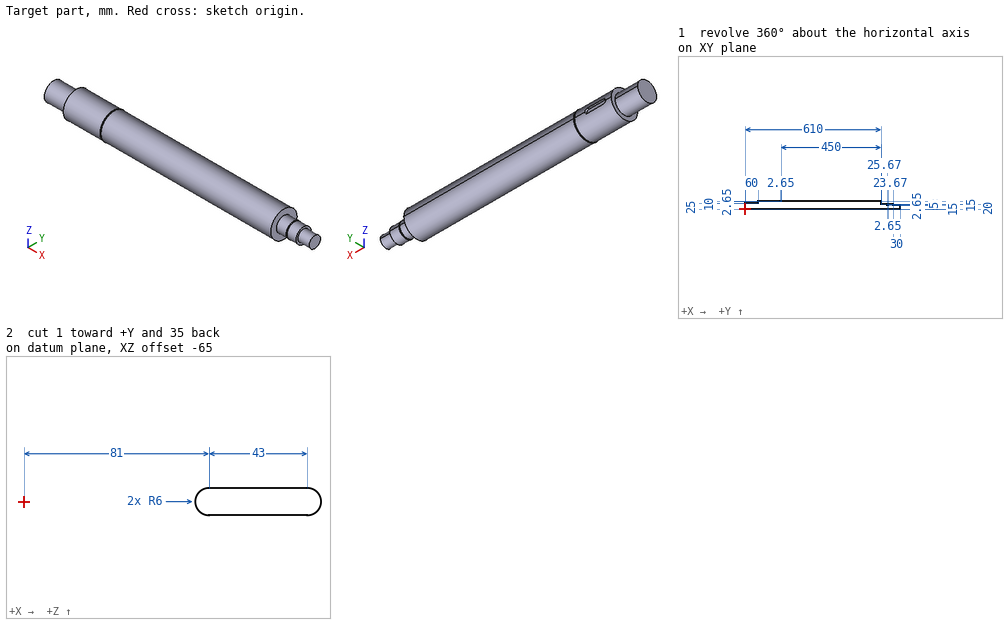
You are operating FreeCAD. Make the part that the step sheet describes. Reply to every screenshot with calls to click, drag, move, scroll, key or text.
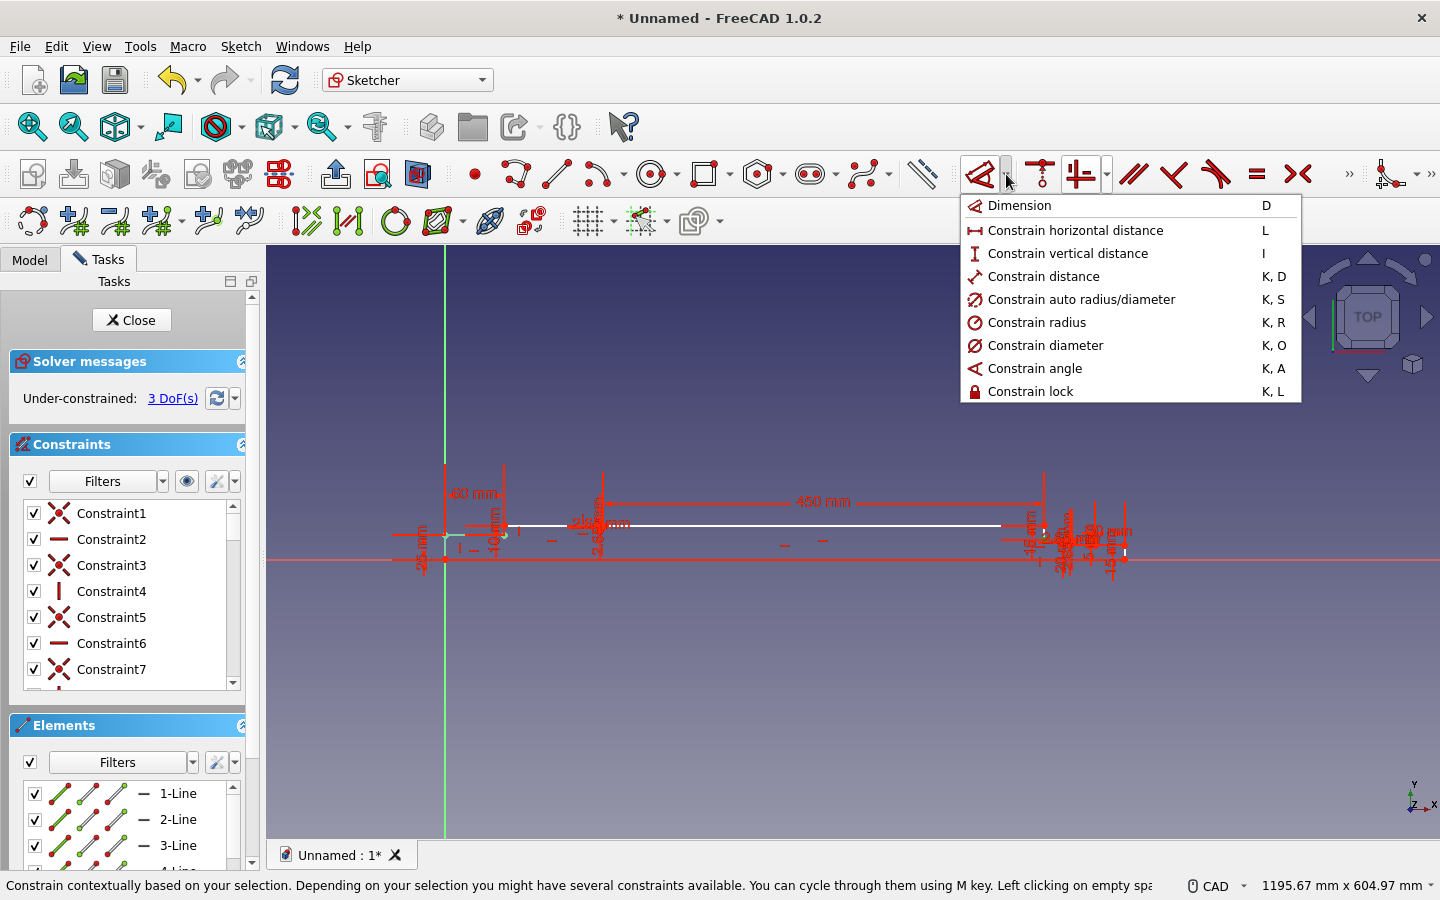
click(1131, 230)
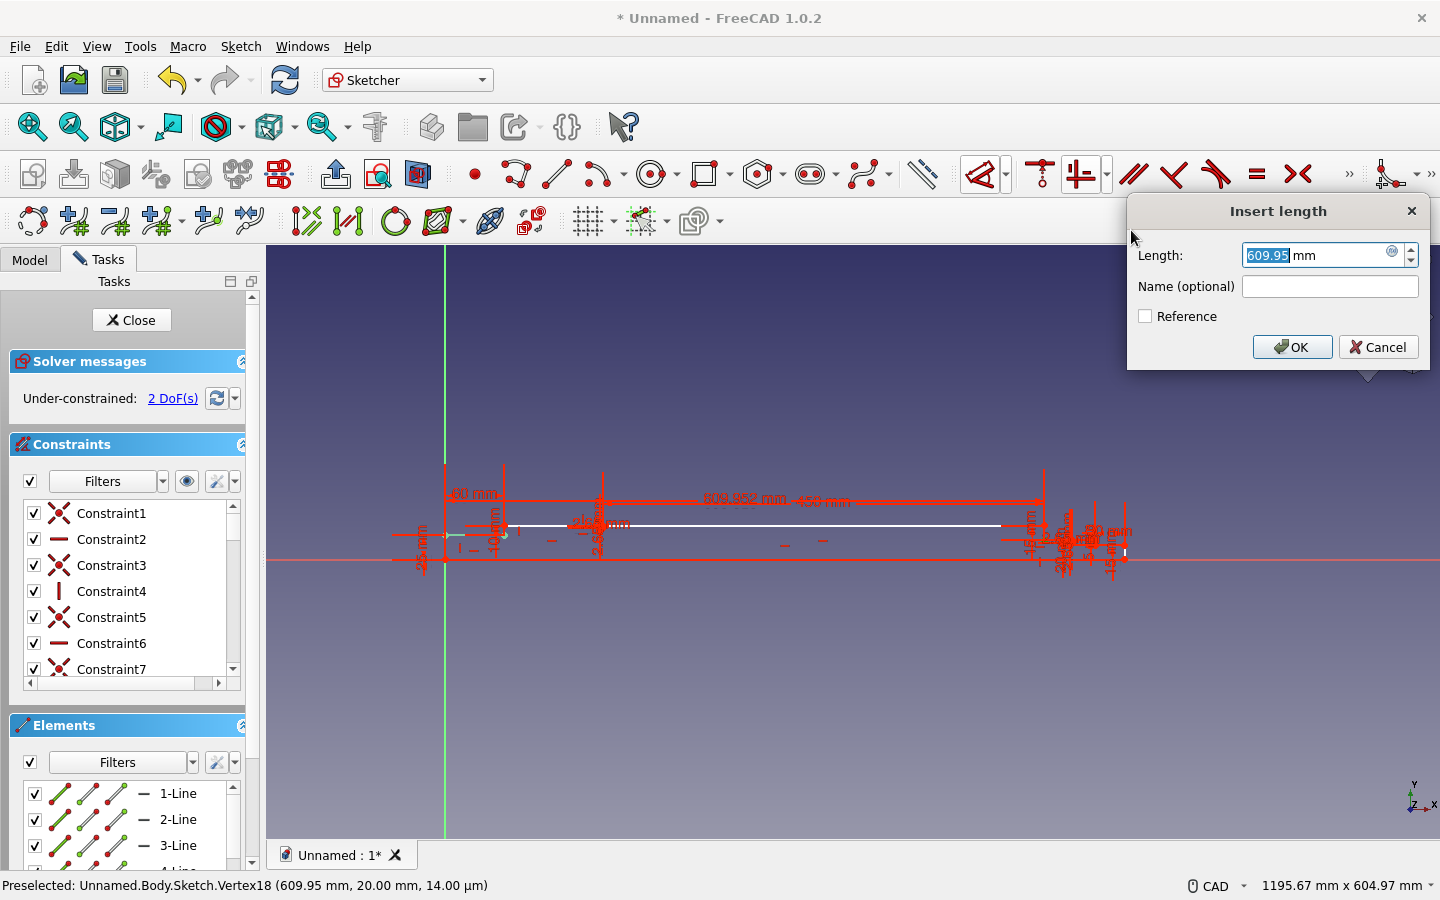
text(610)
key(Return)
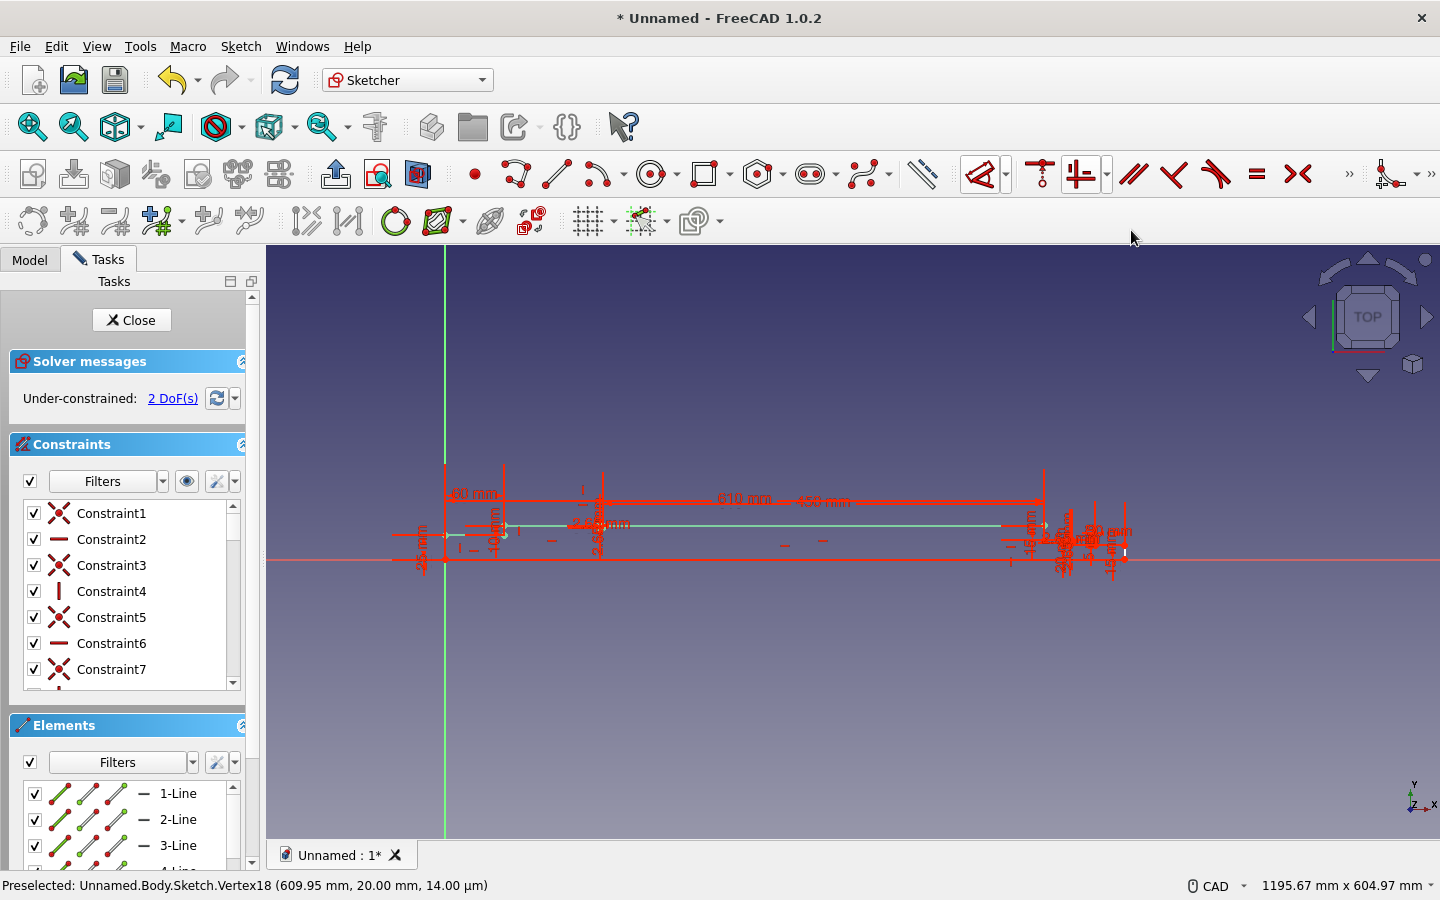
scroll(1086, 540, up, 3)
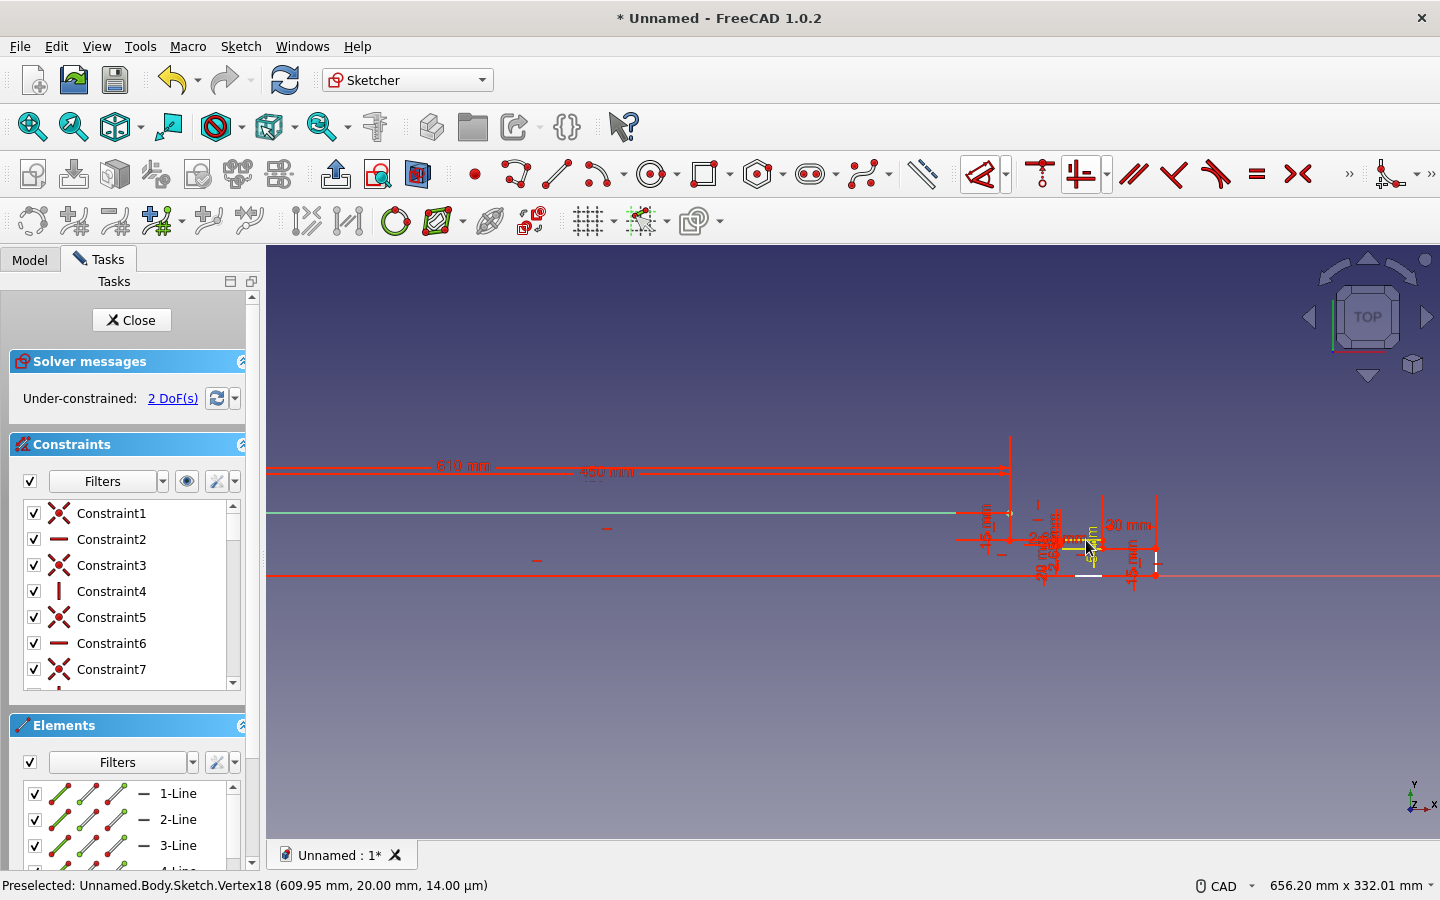
scroll(1085, 540, up, 4)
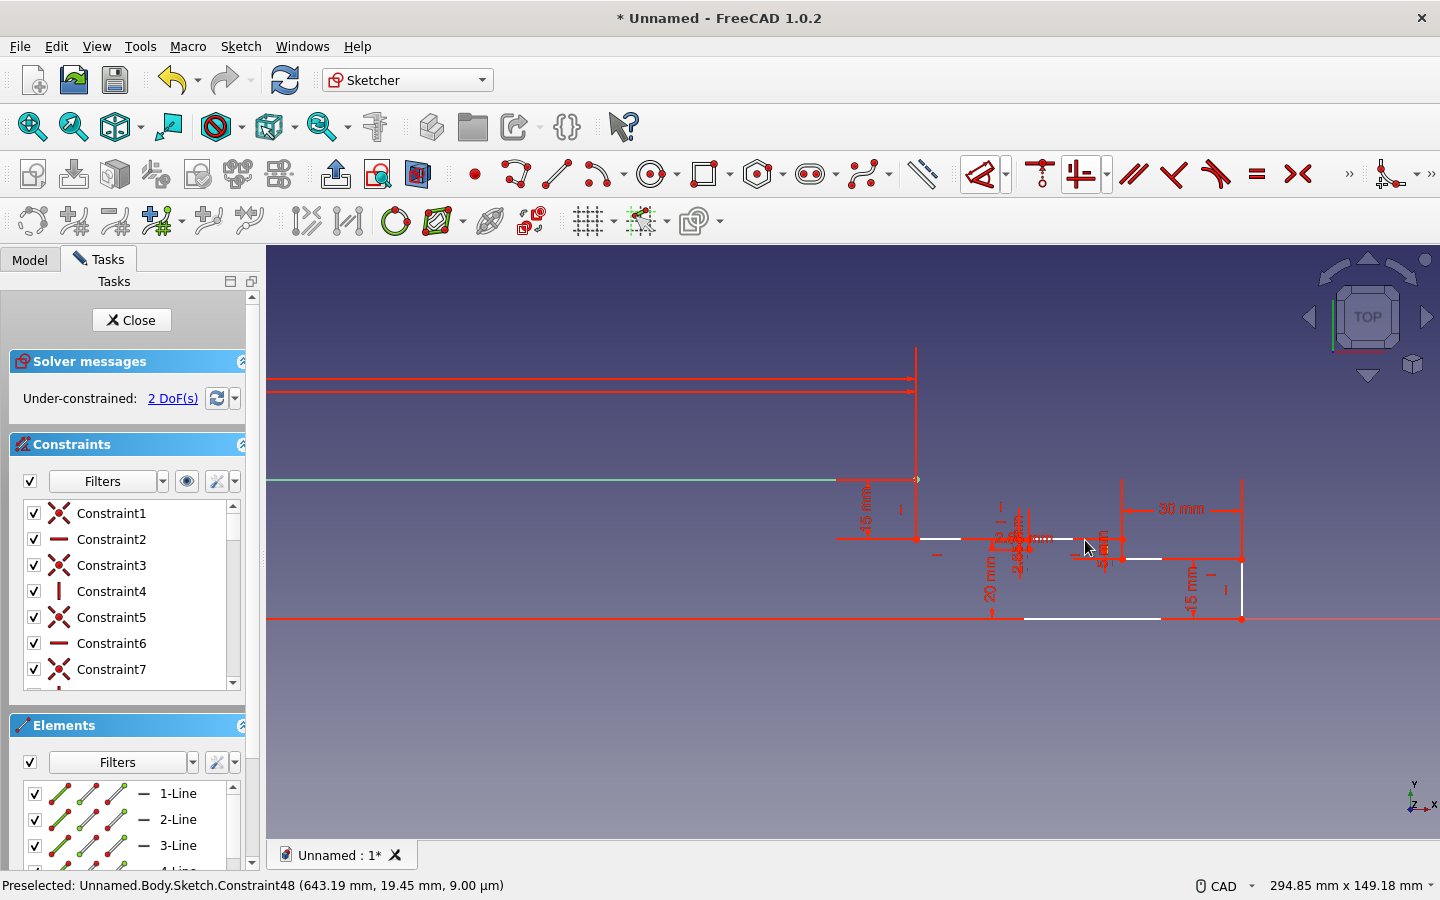
click(1085, 539)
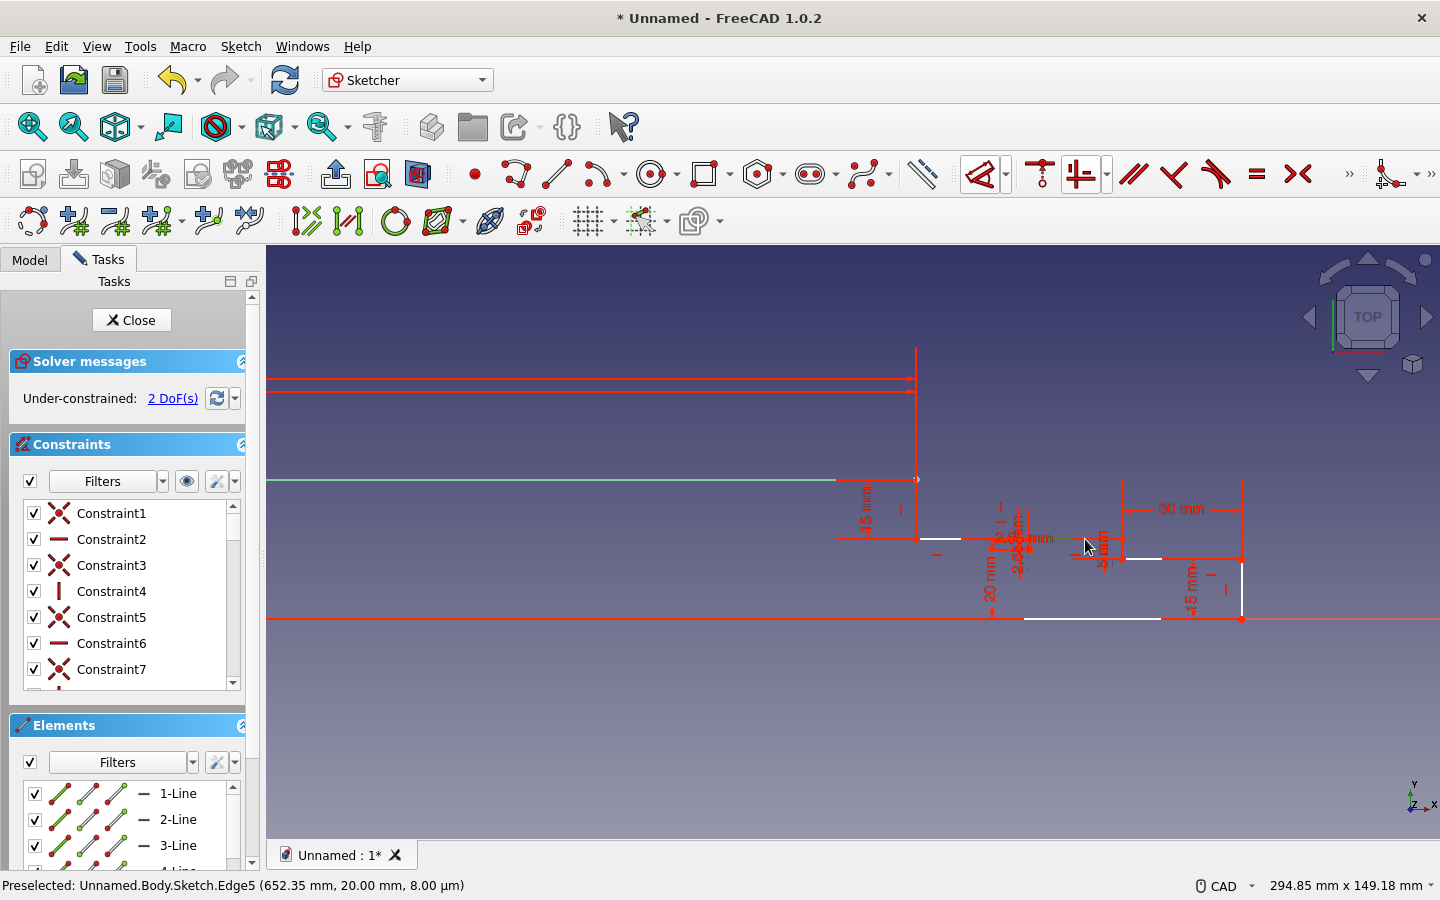
click(1006, 174)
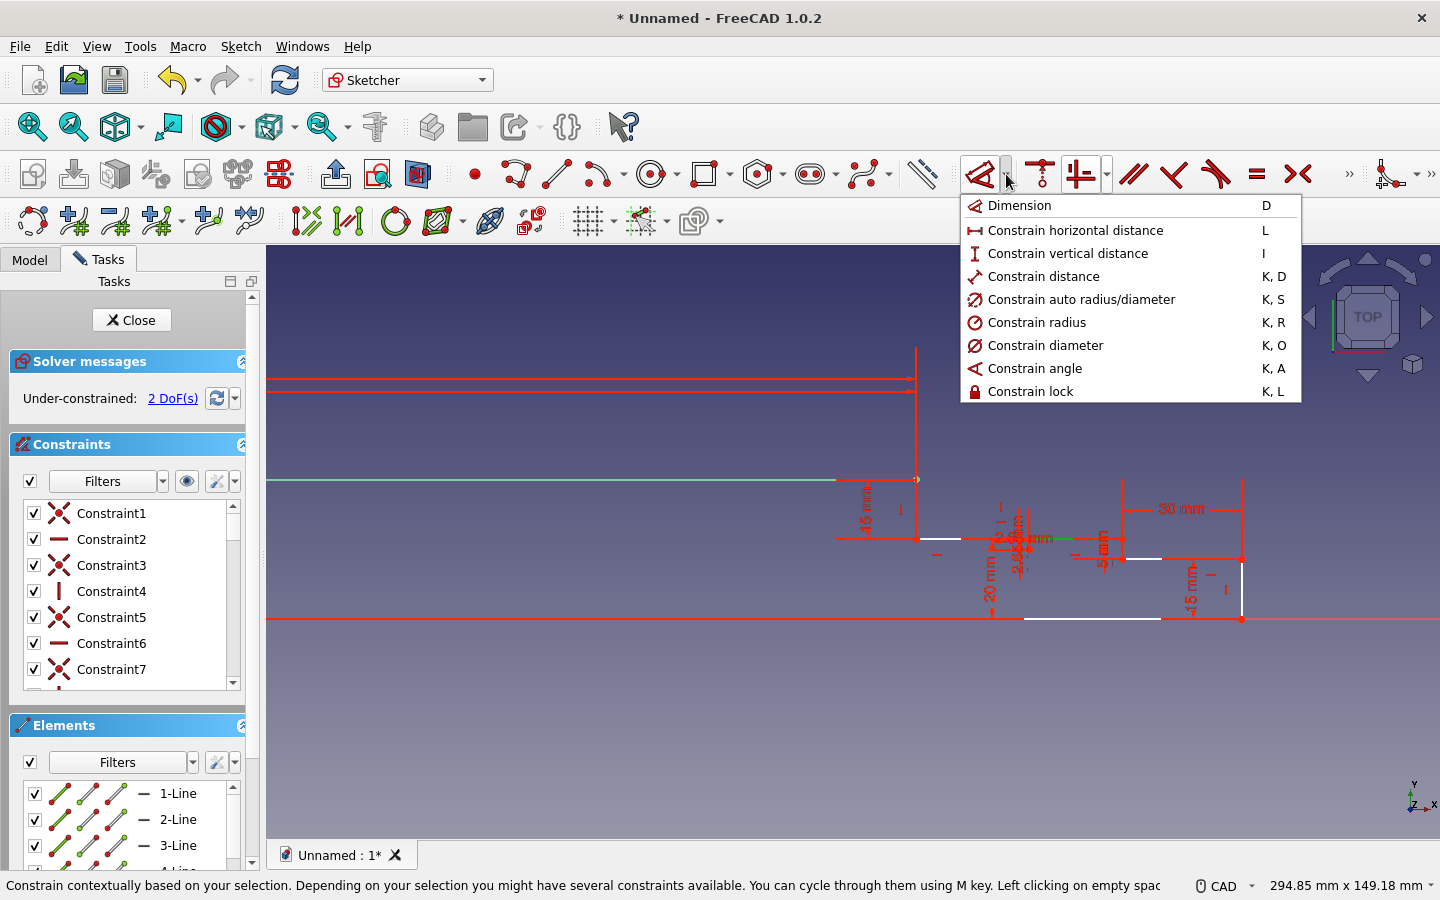
click(1131, 230)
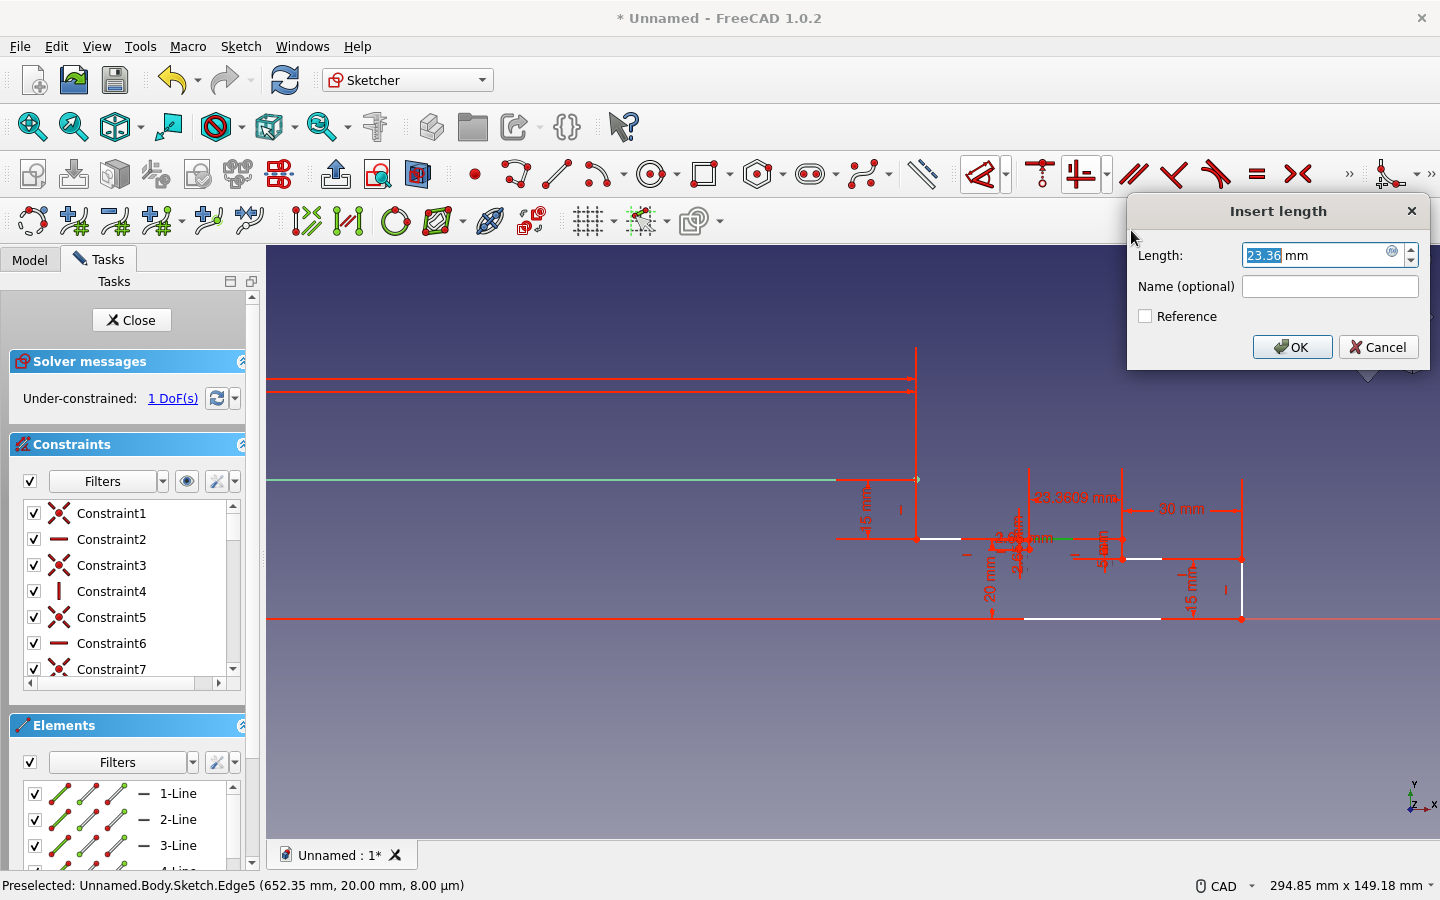
text(23.67)
key(Return)